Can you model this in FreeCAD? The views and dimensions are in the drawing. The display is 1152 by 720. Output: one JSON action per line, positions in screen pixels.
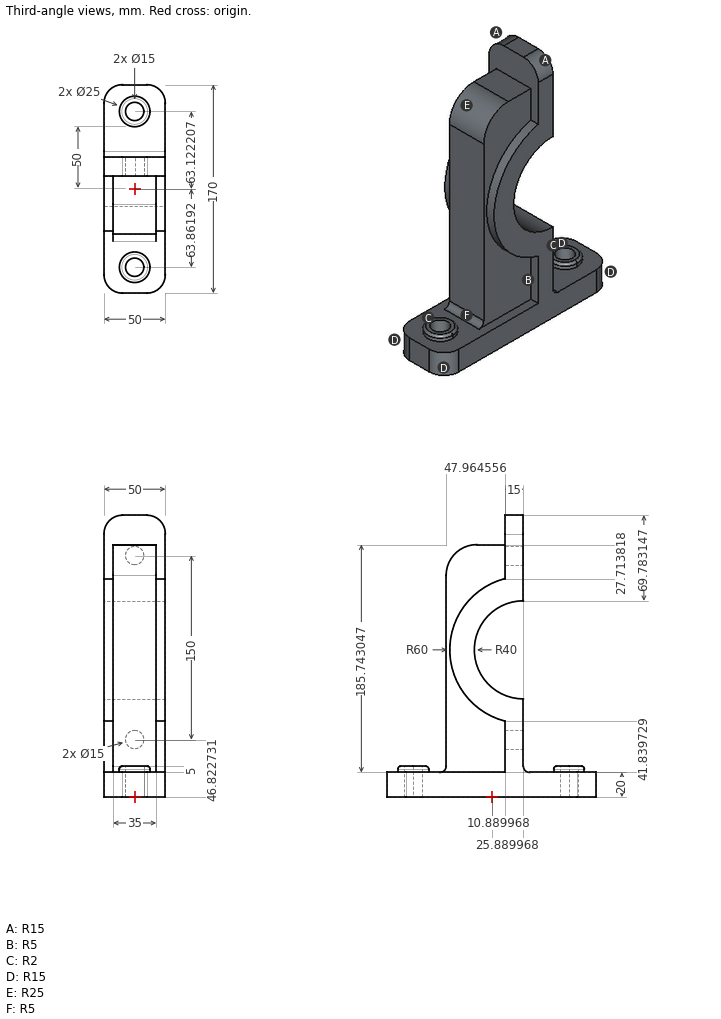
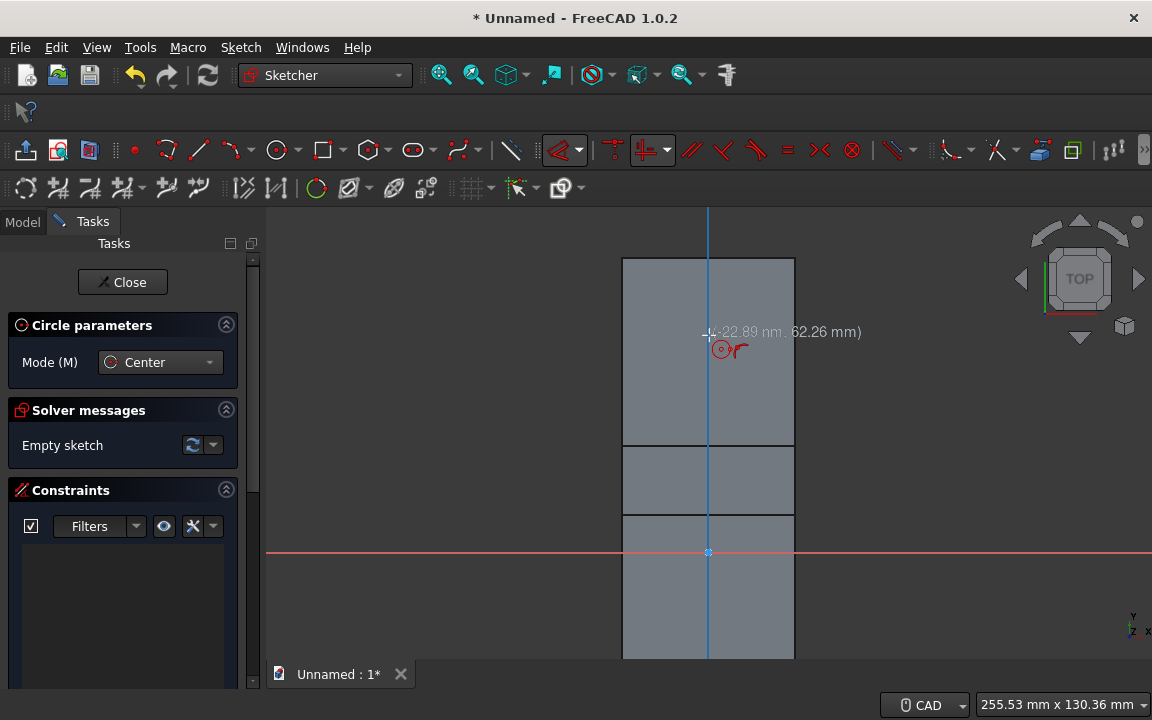
{"action": "left_click", "coordinate": [708, 334]}
{"action": "mouse_move", "coordinate": [727, 316]}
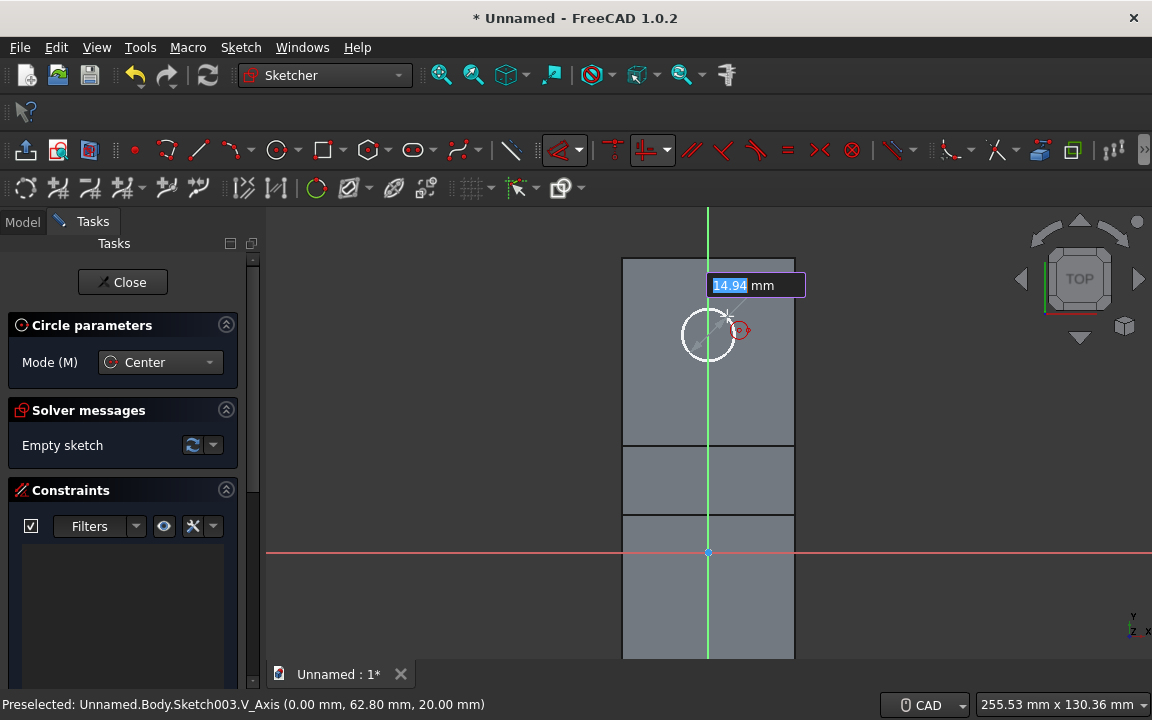
{"action": "type", "text": "15"}
{"action": "key", "text": "Return"}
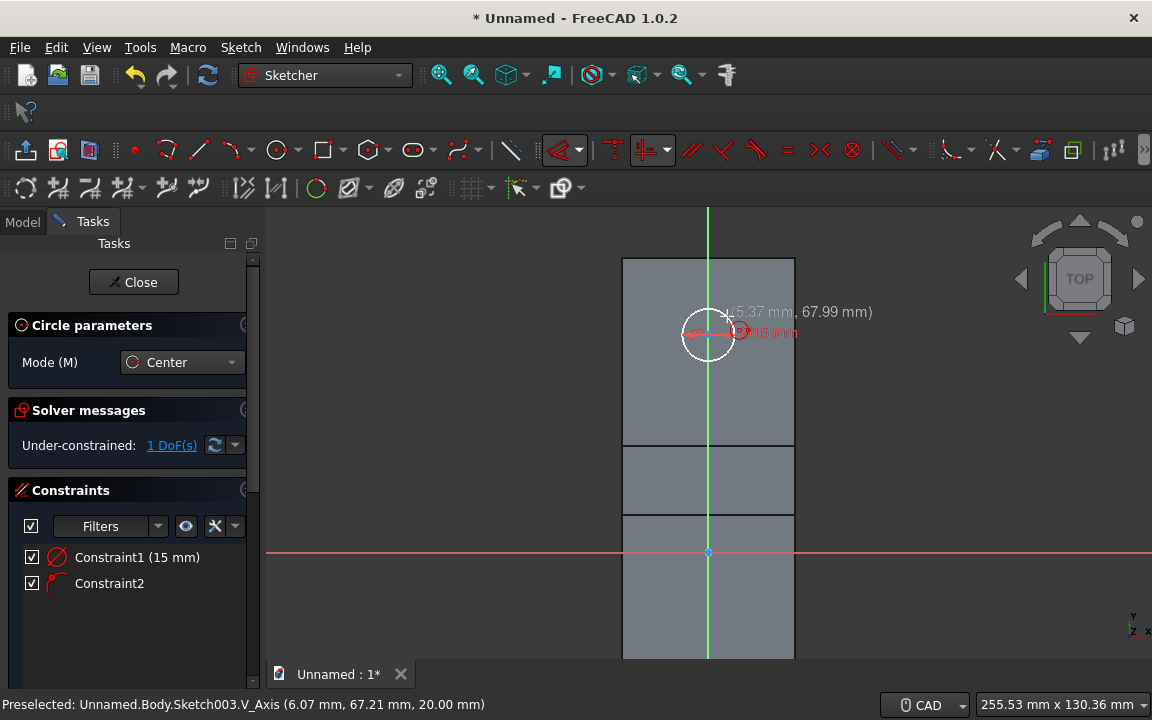
{"action": "scroll", "coordinate": [558, 286], "scroll_direction": "down", "scroll_amount": 3}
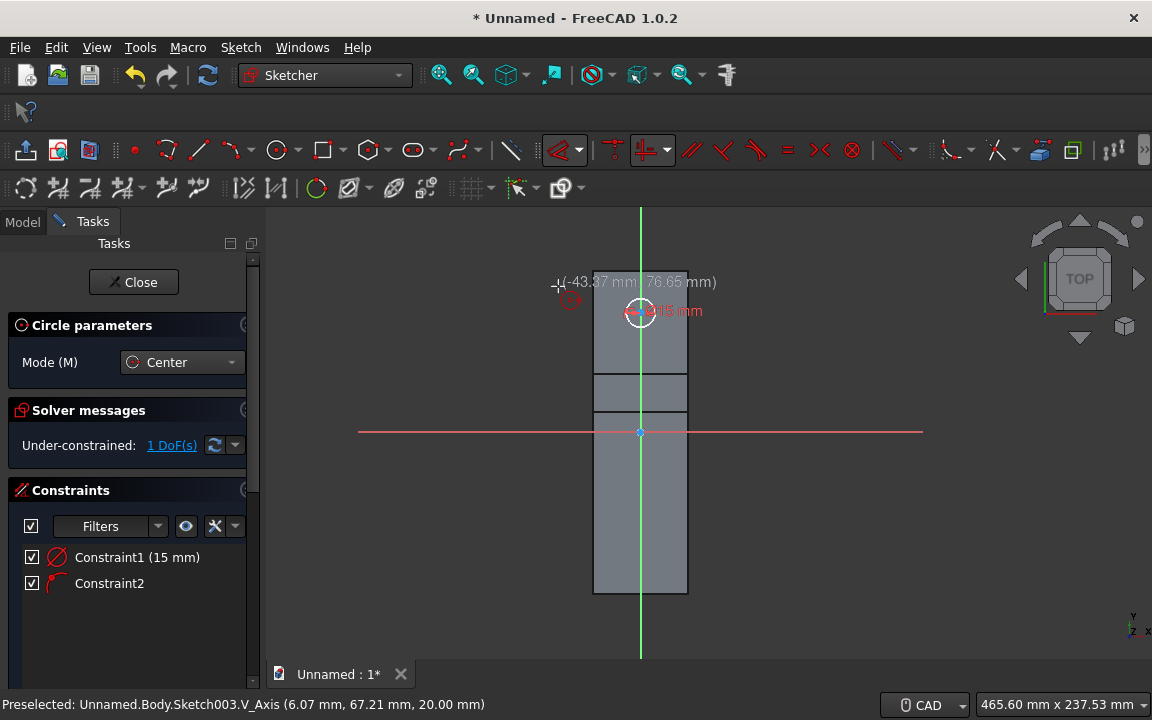
{"action": "scroll", "coordinate": [641, 554], "scroll_direction": "up", "scroll_amount": 3}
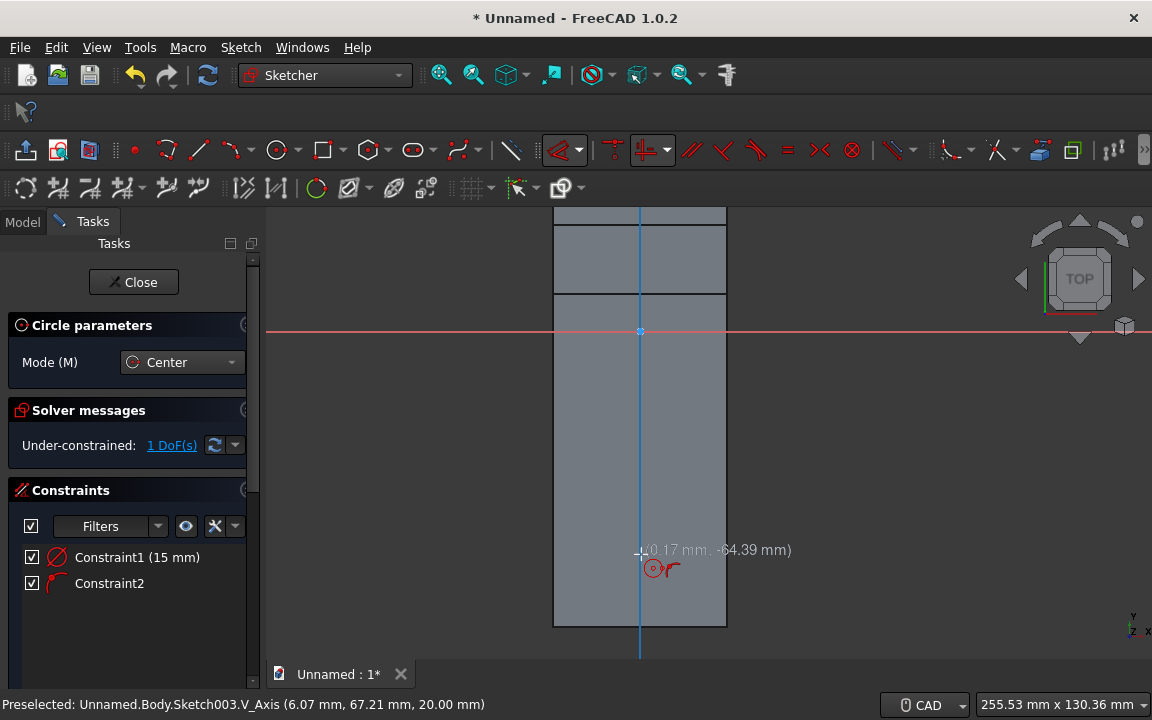
{"action": "left_click", "coordinate": [640, 553]}
{"action": "mouse_move", "coordinate": [658, 535]}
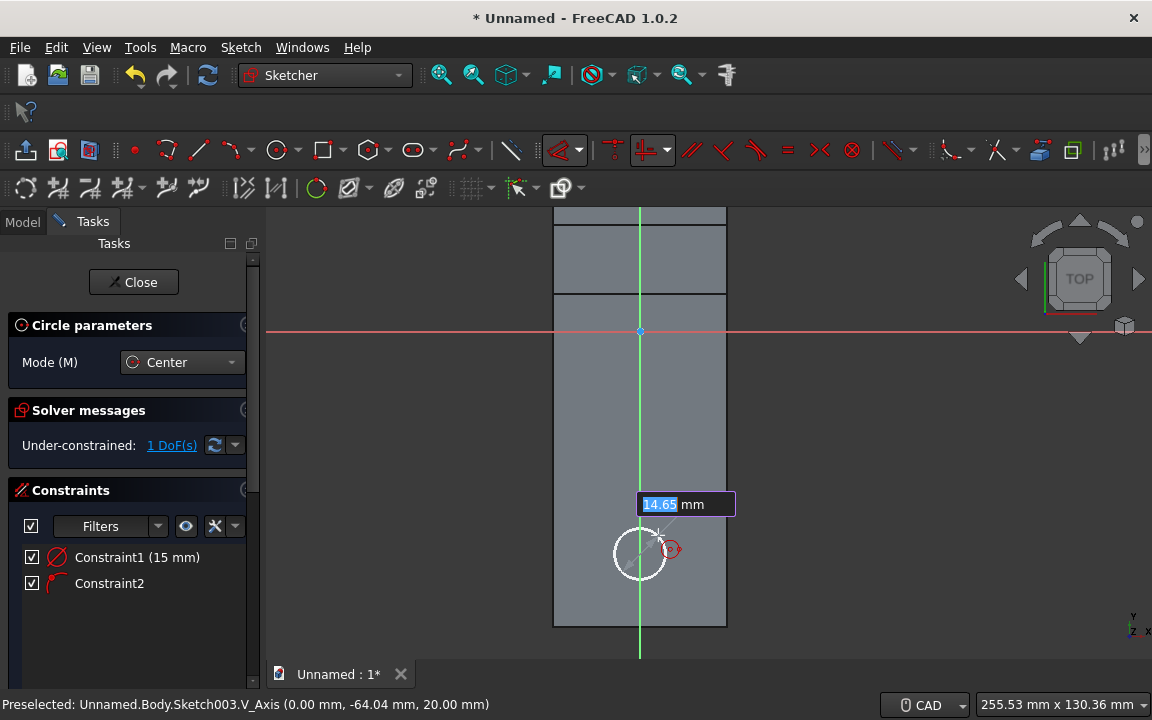
{"action": "type", "text": "15"}
{"action": "key", "text": "Return"}
{"action": "key", "text": "Escape"}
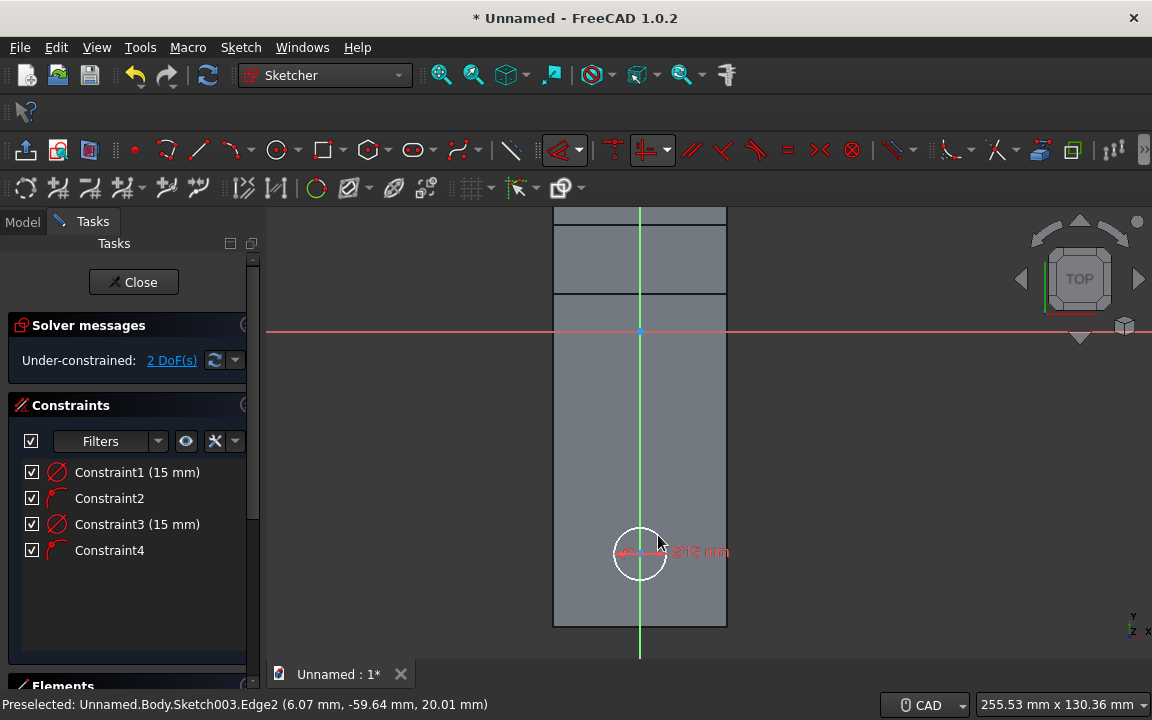
{"action": "left_click", "coordinate": [640, 554]}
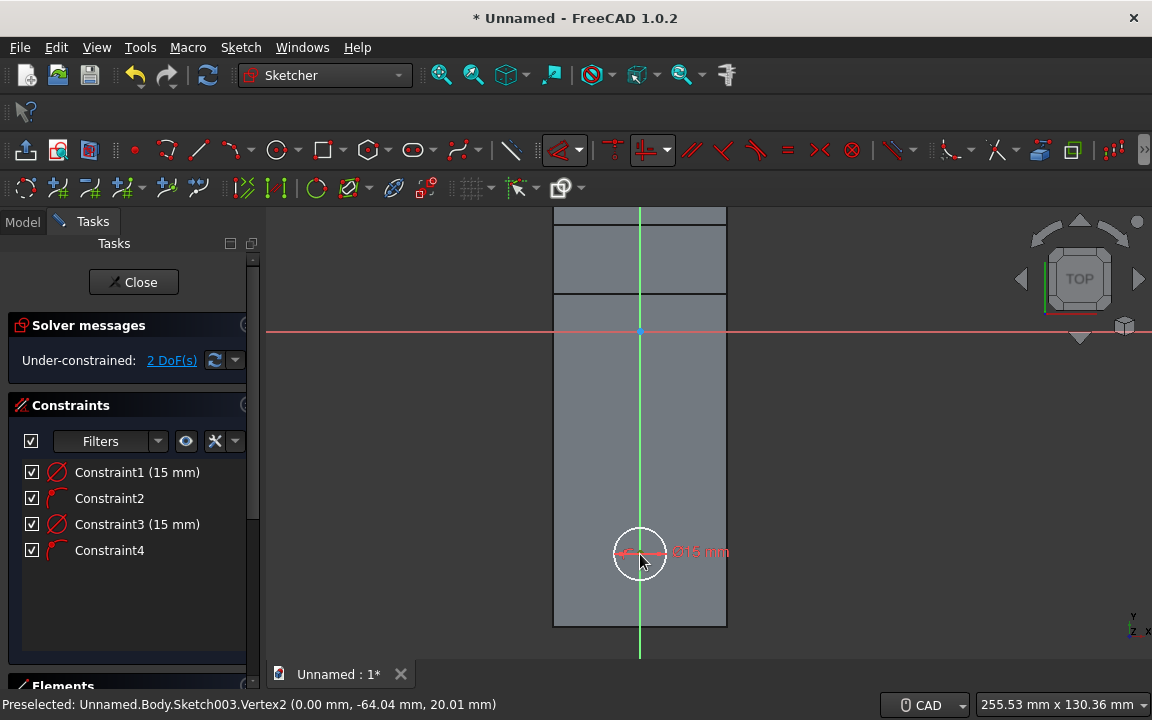
{"action": "left_click", "coordinate": [582, 150]}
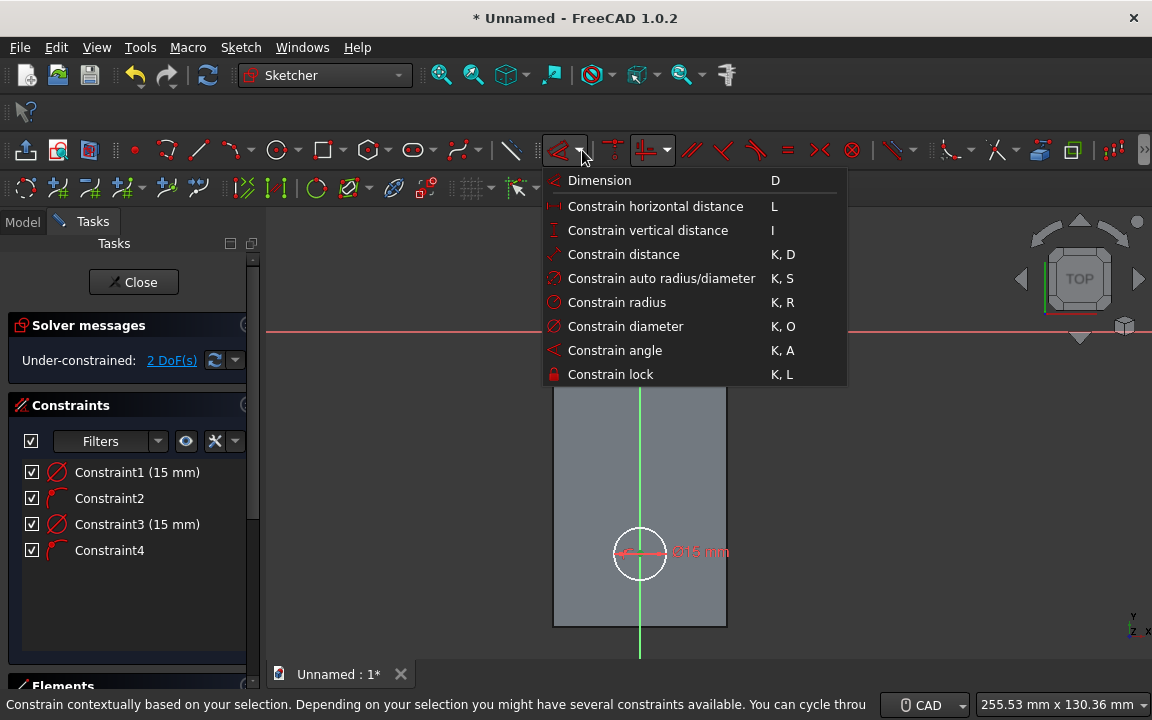
{"action": "left_click", "coordinate": [695, 230]}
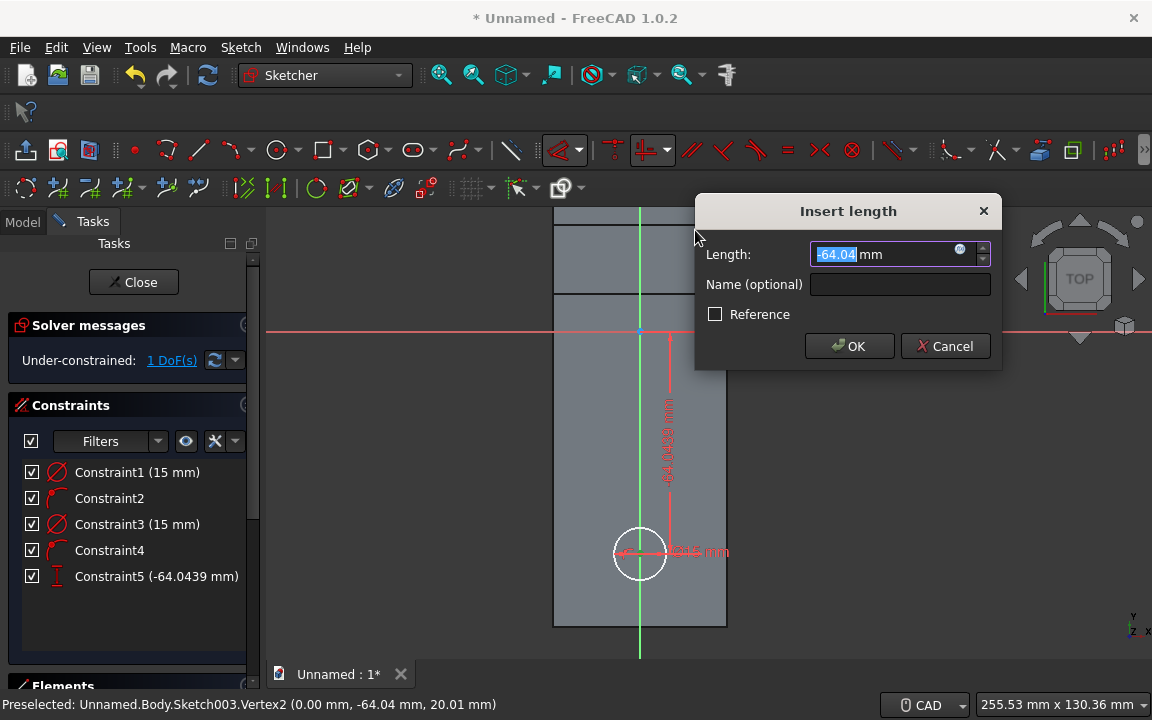
{"action": "type", "text": "-63.86192"}
{"action": "key", "text": "Return"}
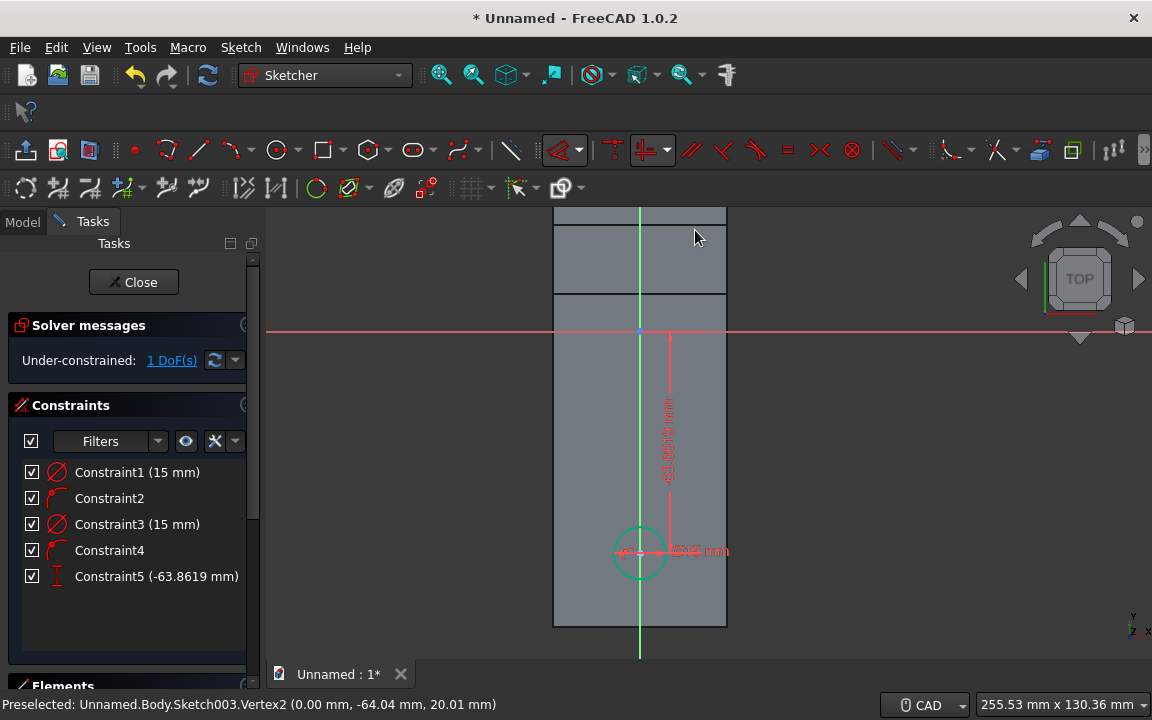
{"action": "scroll", "coordinate": [641, 554], "scroll_direction": "down", "scroll_amount": 3}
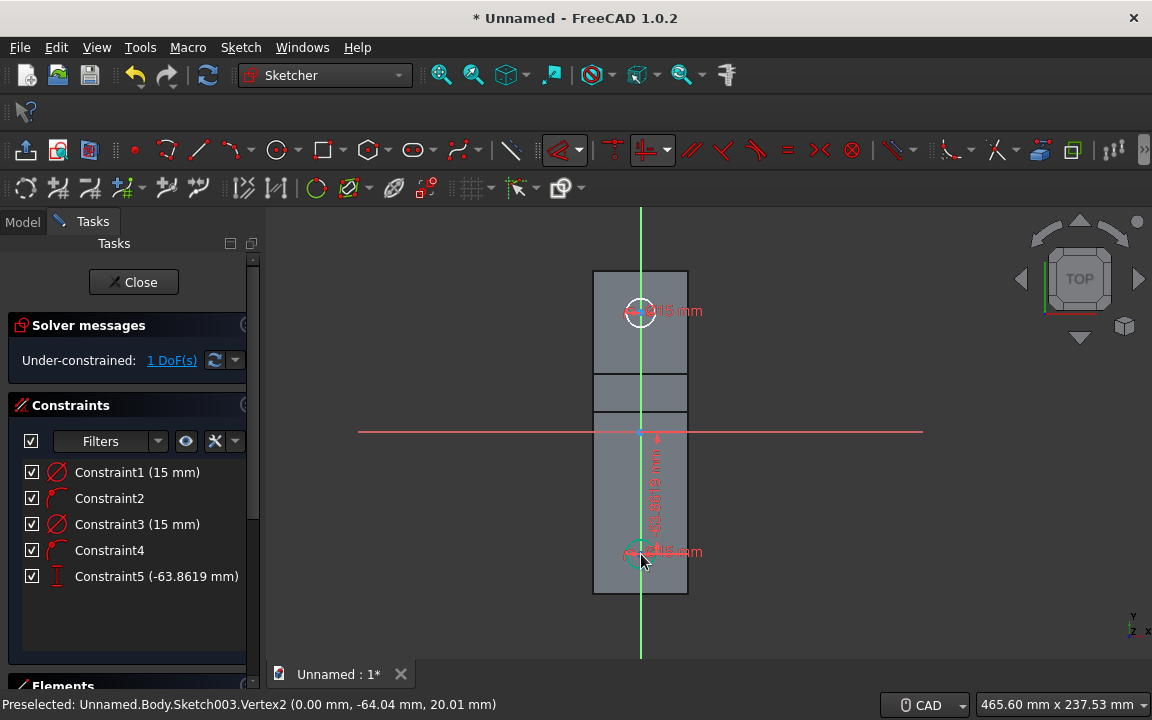
{"action": "left_click", "coordinate": [641, 313]}